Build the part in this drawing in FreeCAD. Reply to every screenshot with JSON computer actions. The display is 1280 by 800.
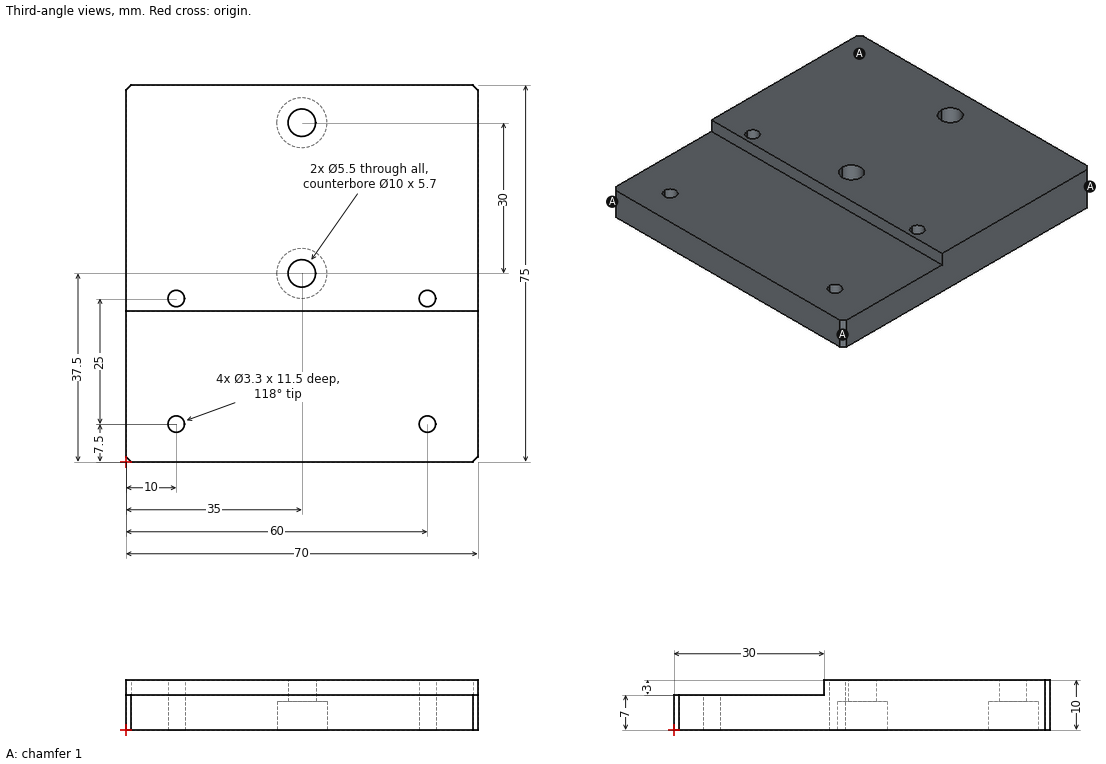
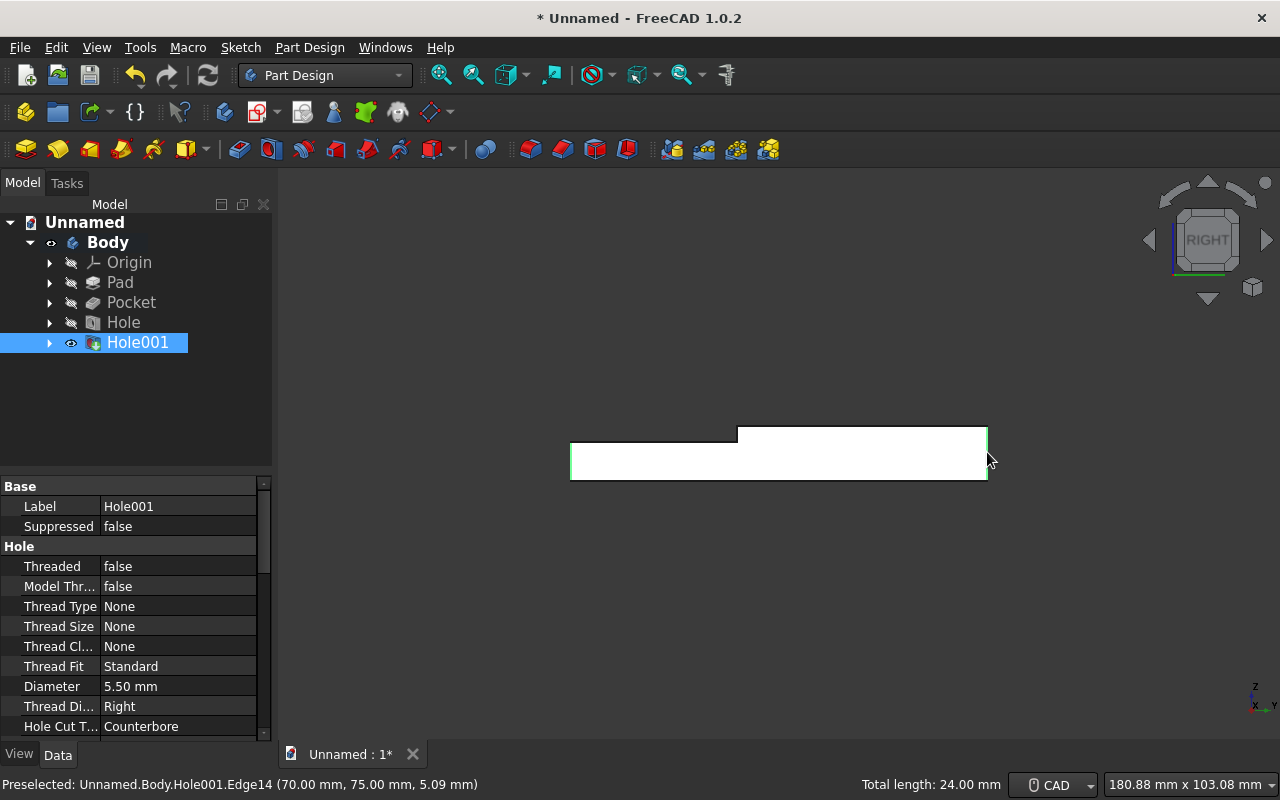
{"action": "key", "text": "5"}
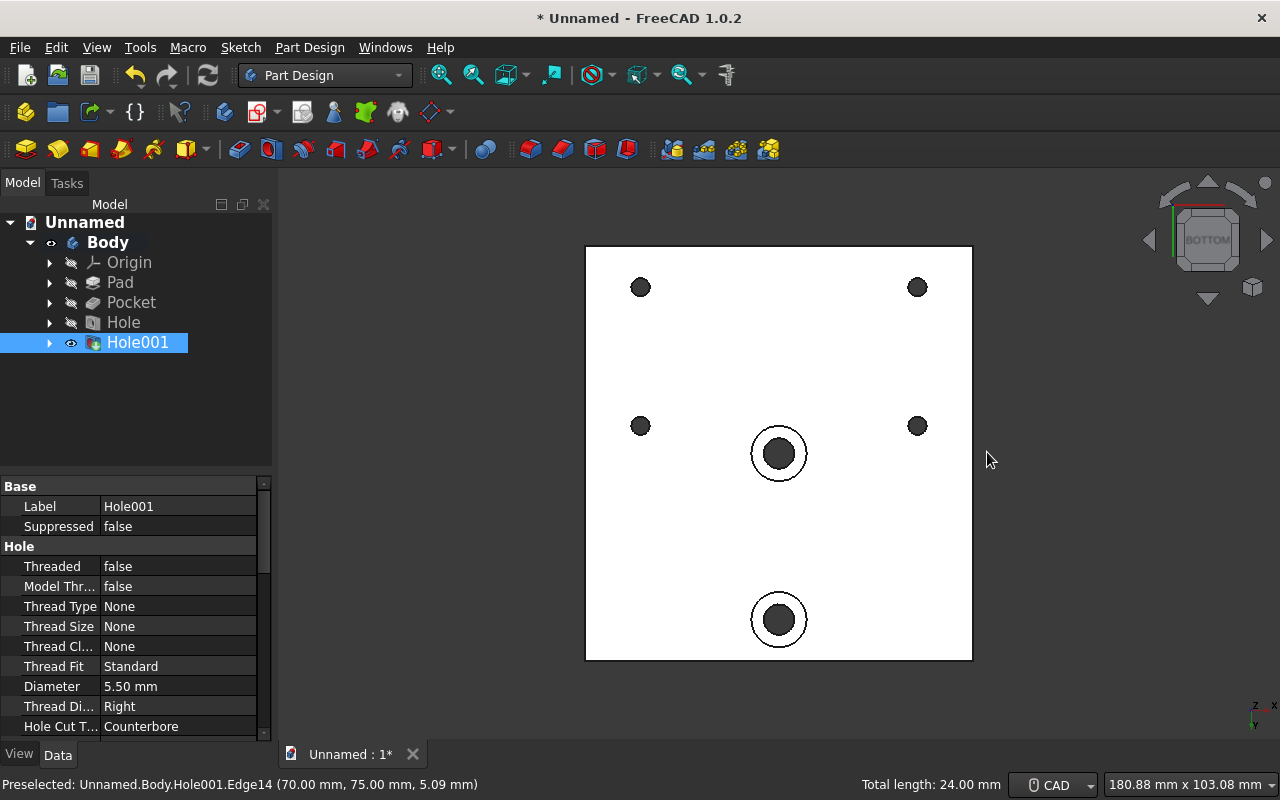
{"action": "key", "text": "4"}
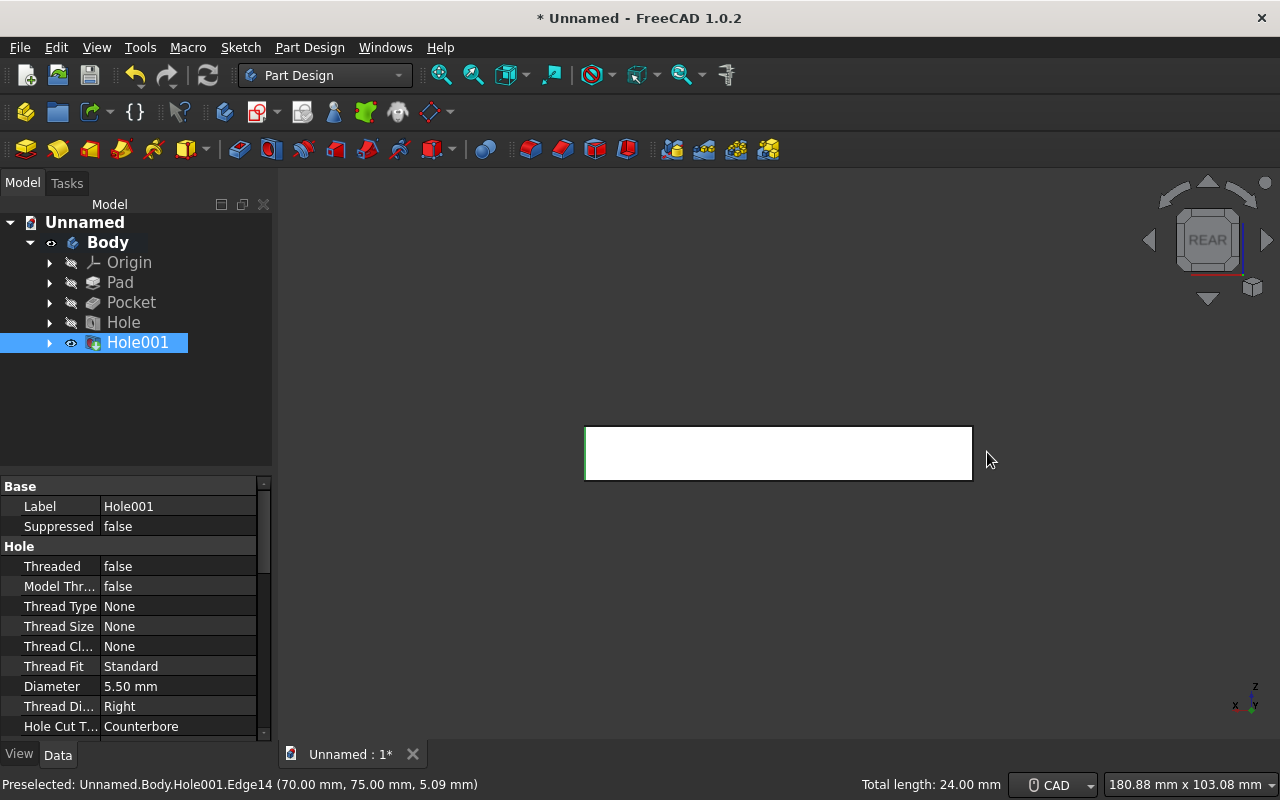
{"action": "left_click", "coordinate": [442, 76]}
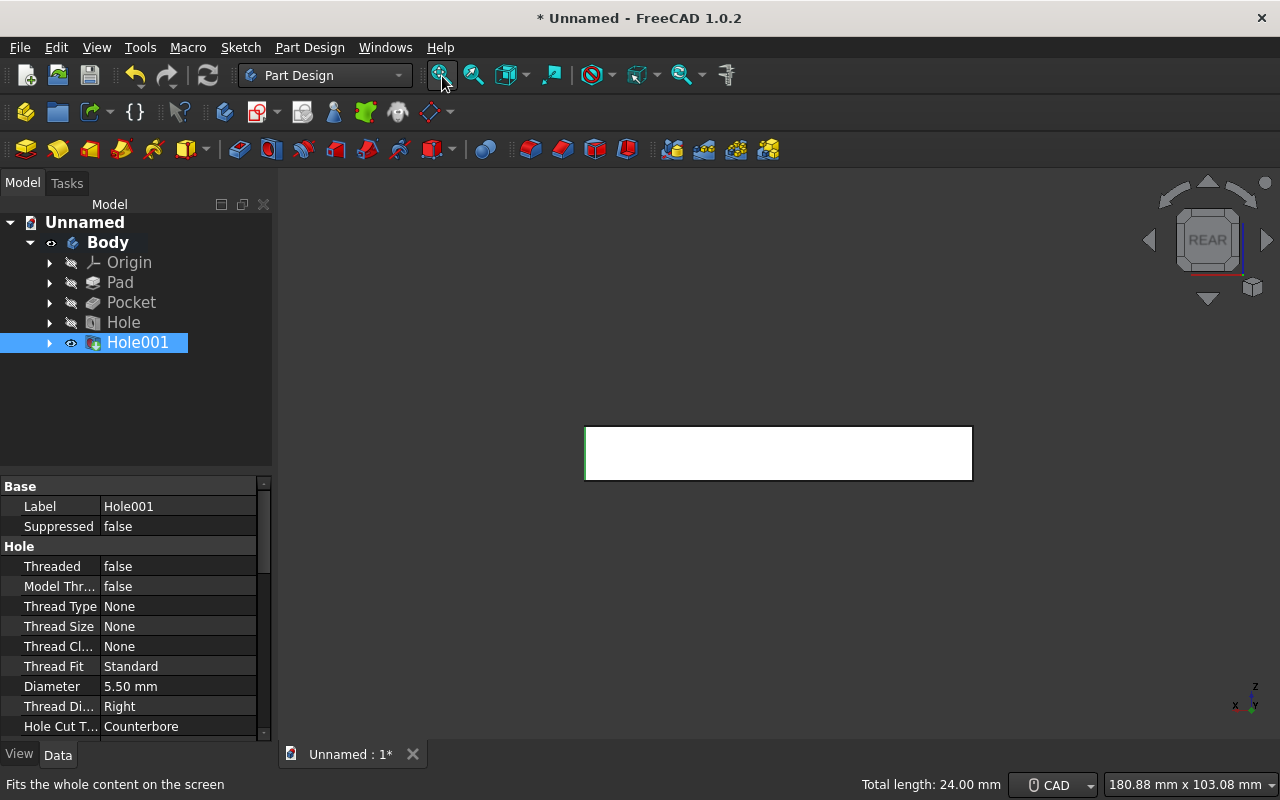
{"action": "left_click", "coordinate": [973, 453], "text": "ctrl"}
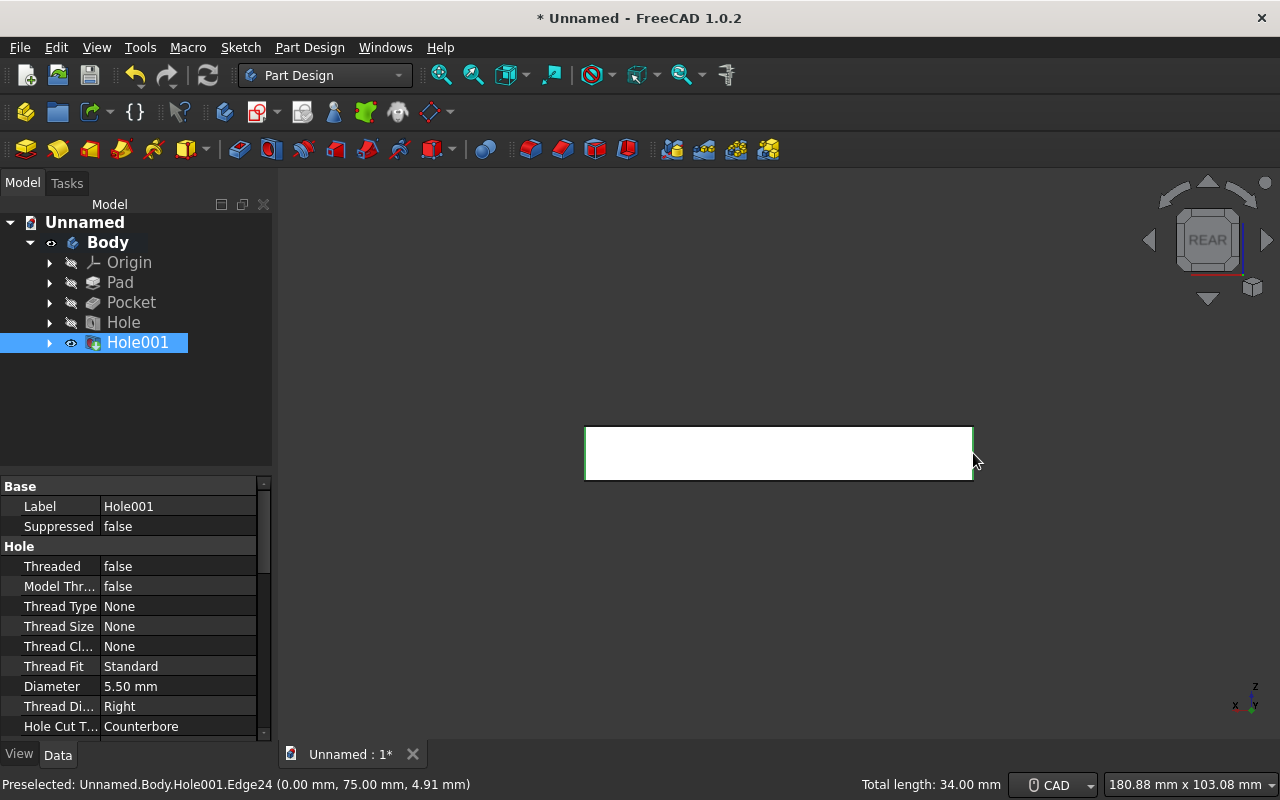
{"action": "left_click", "coordinate": [564, 150]}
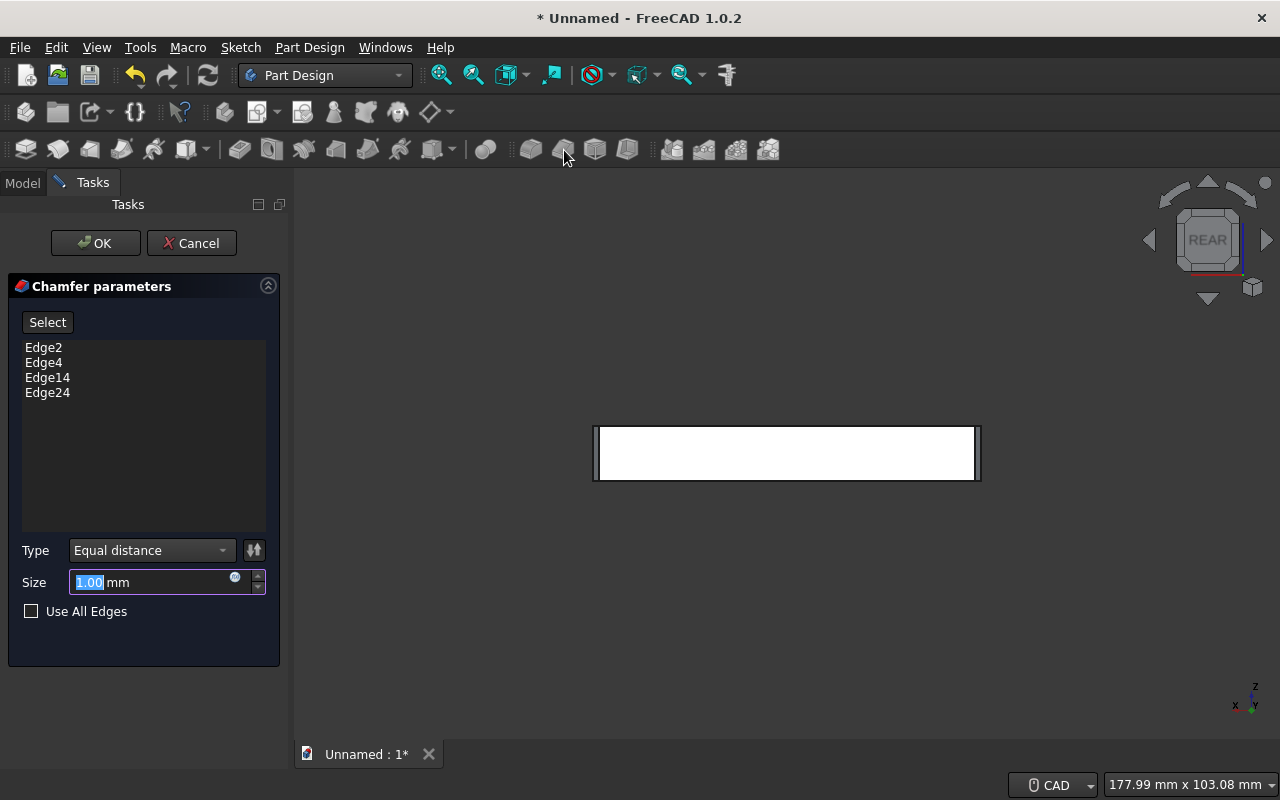
{"action": "type", "text": "1"}
{"action": "key", "text": "Tab"}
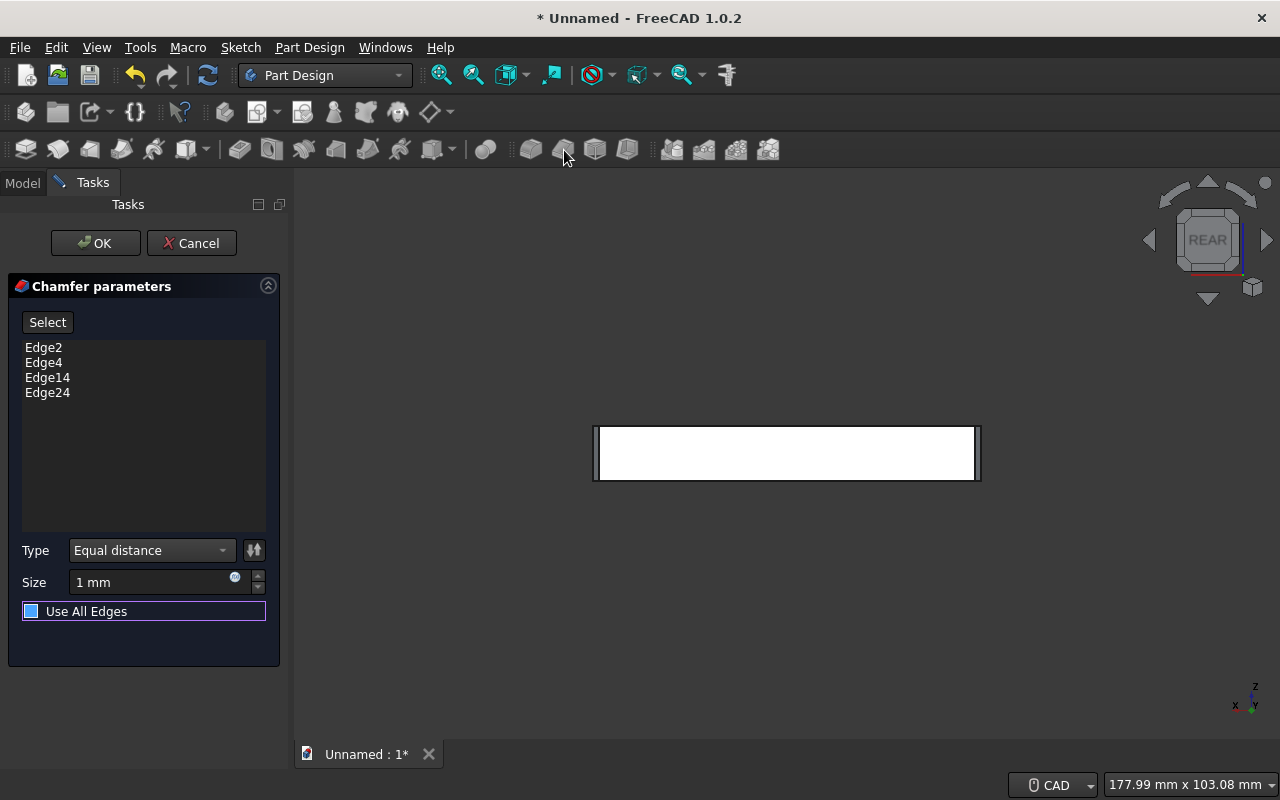
{"action": "left_click", "coordinate": [96, 243]}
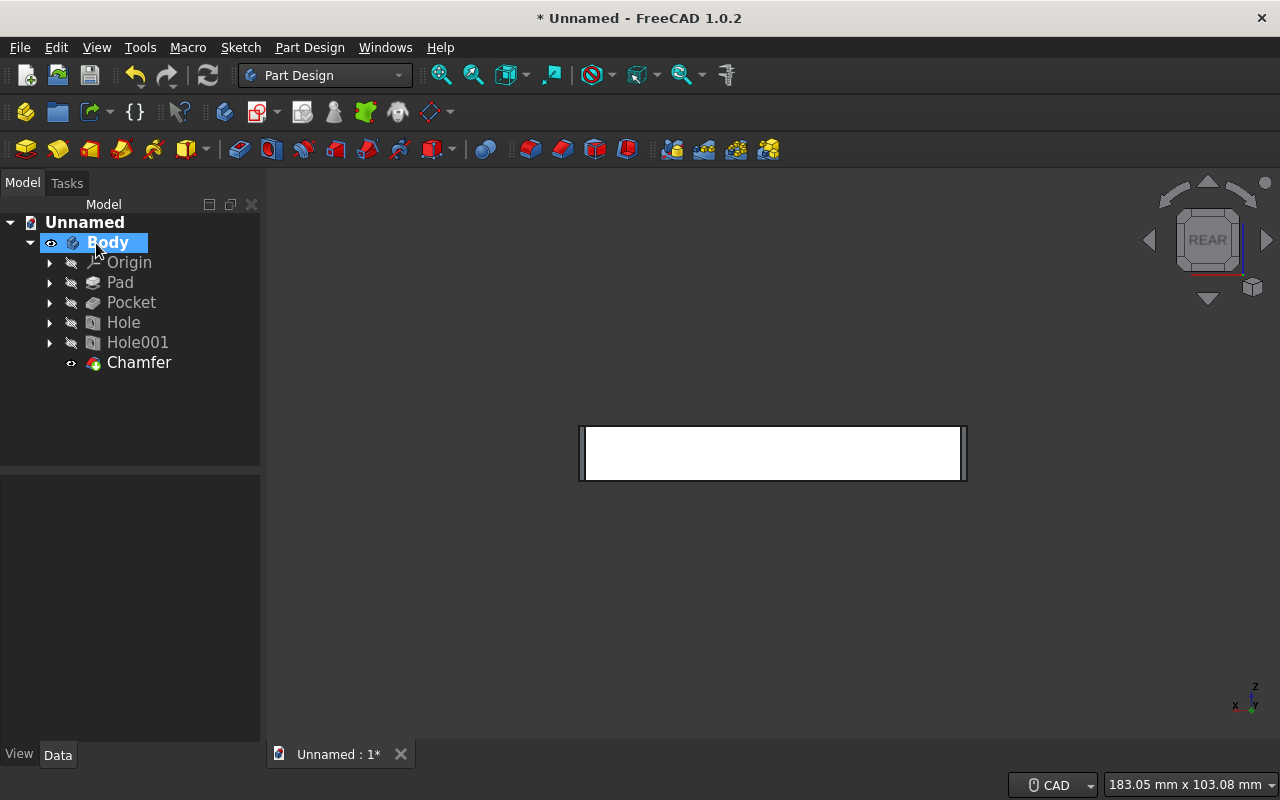
{"action": "key", "text": "0"}